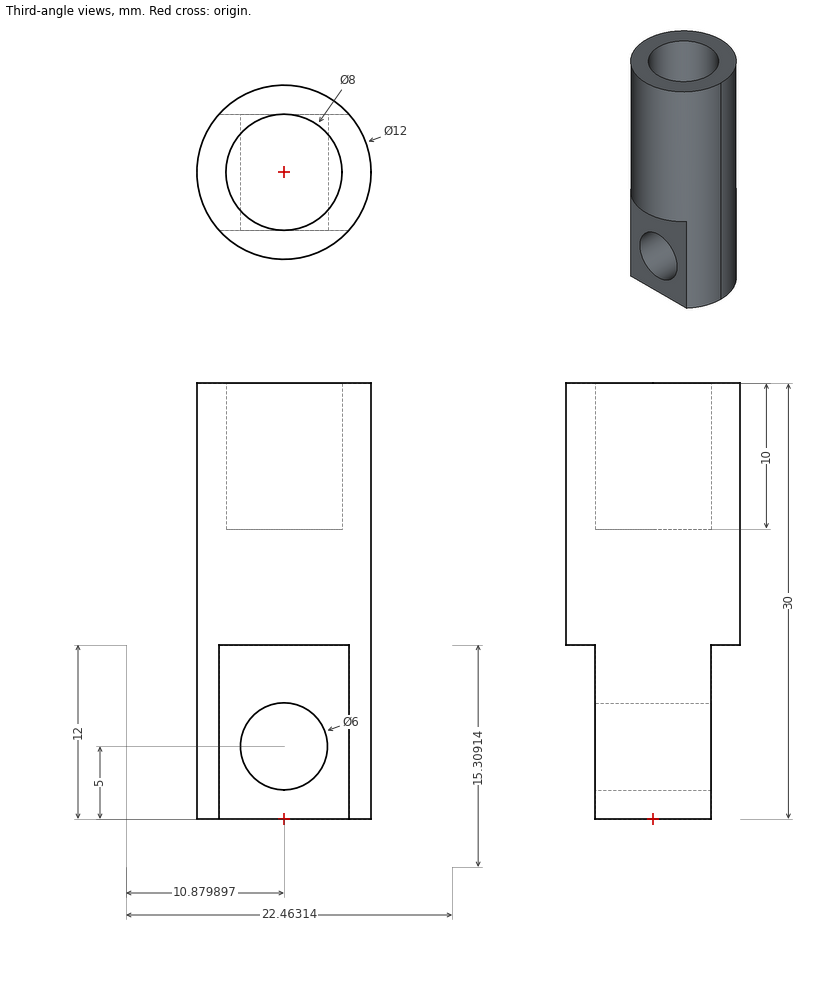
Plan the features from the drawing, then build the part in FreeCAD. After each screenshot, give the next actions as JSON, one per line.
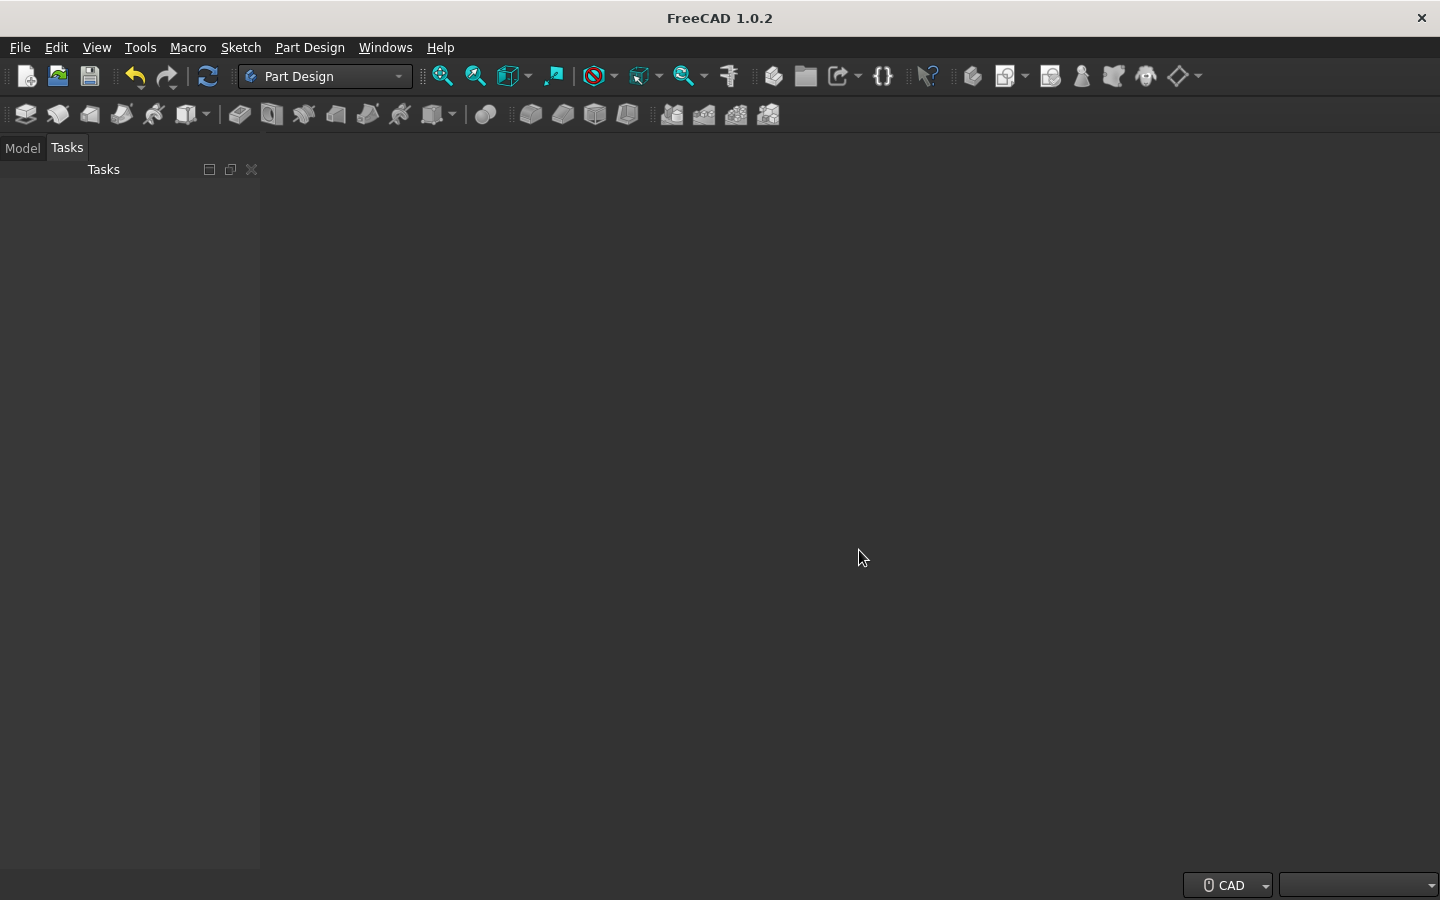
{"action": "left_click", "coordinate": [26, 76]}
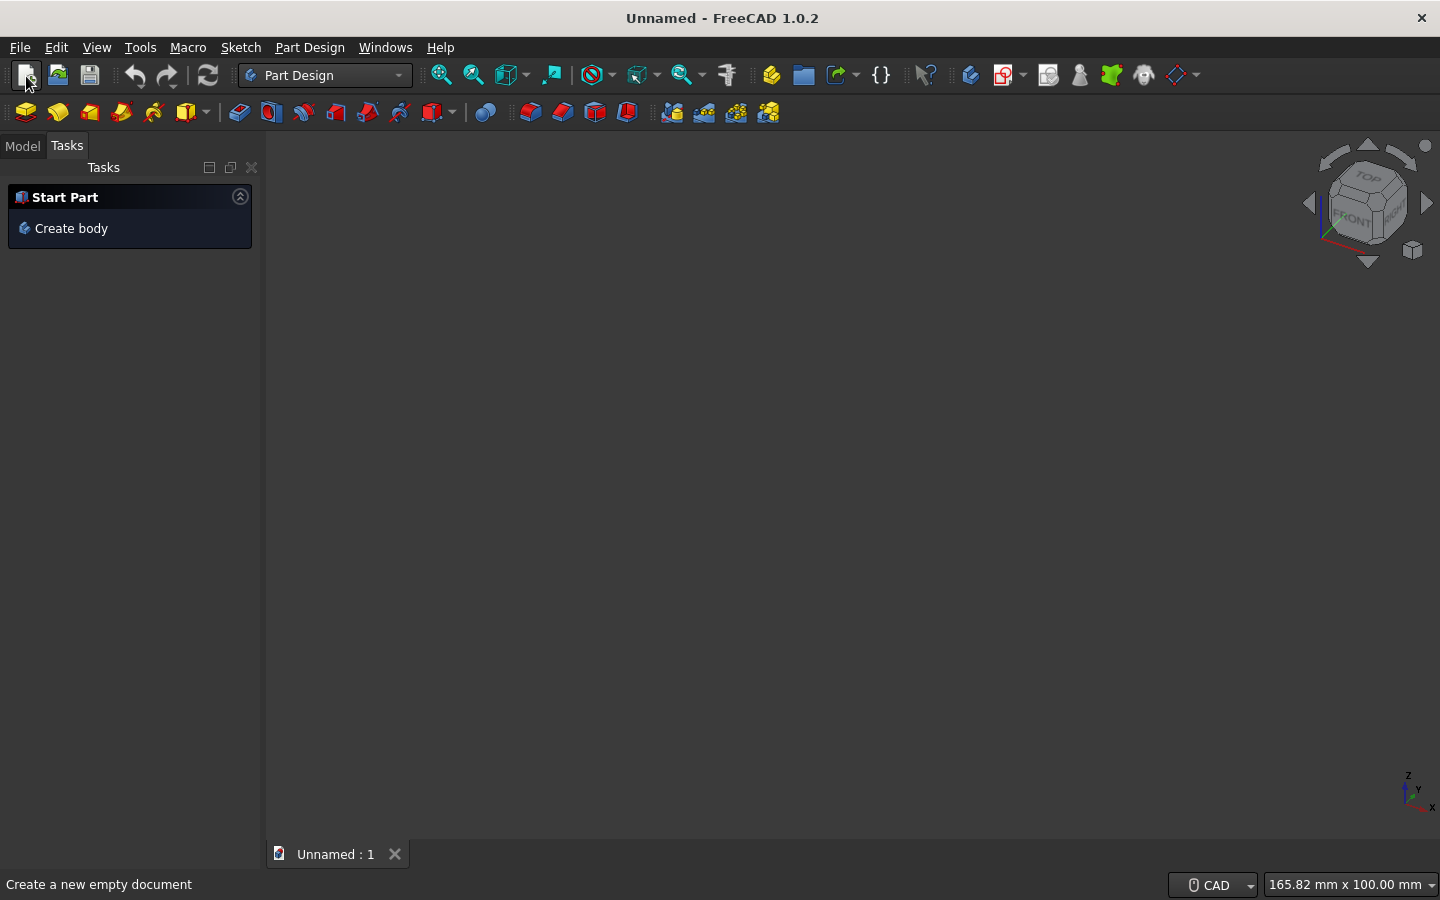
{"action": "left_click", "coordinate": [1004, 76]}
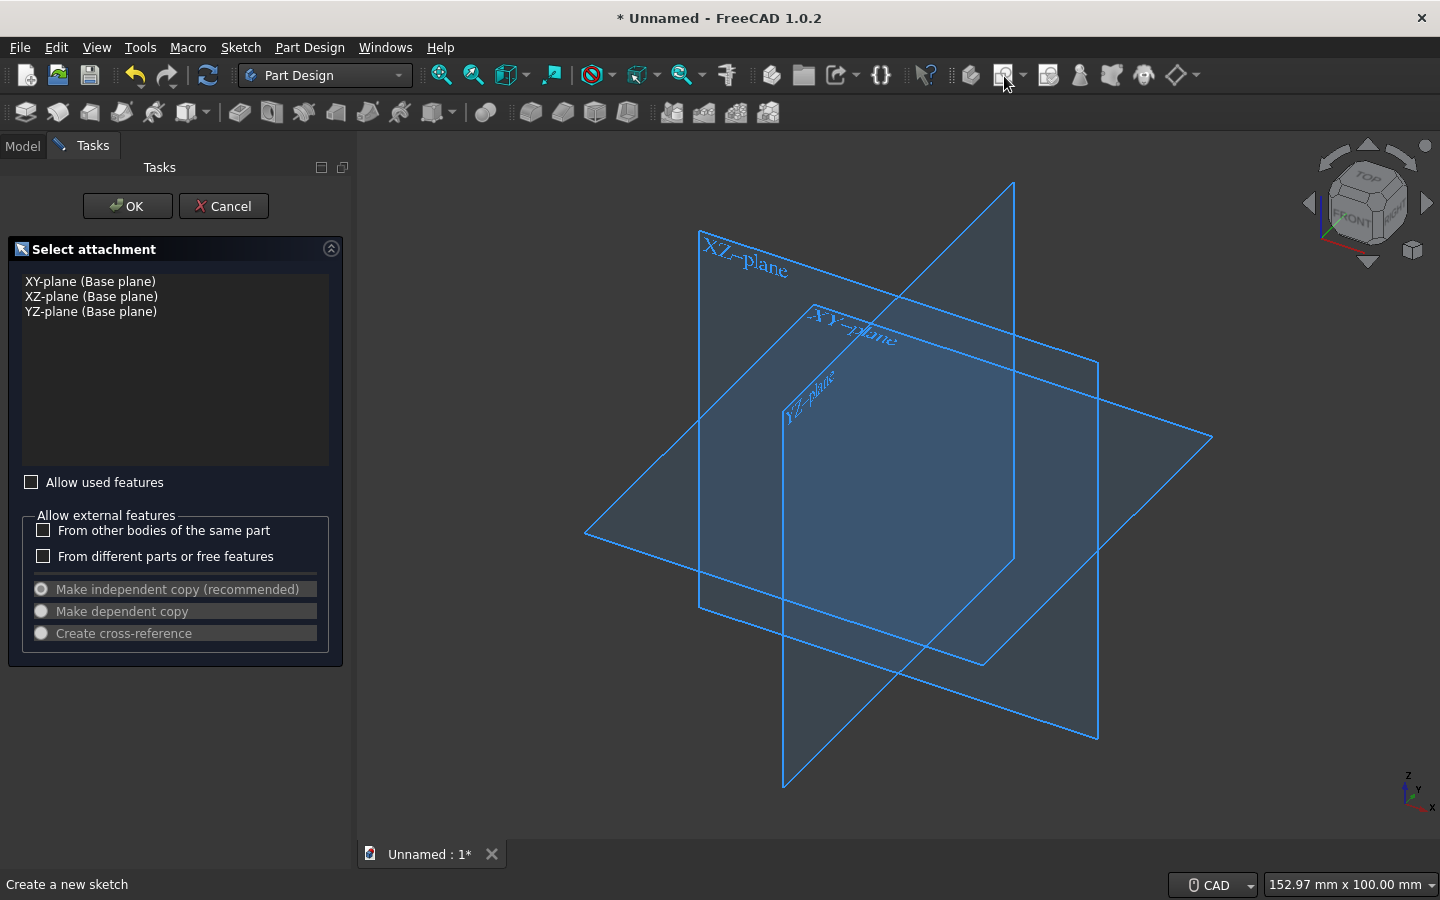
{"action": "left_click", "coordinate": [82, 282]}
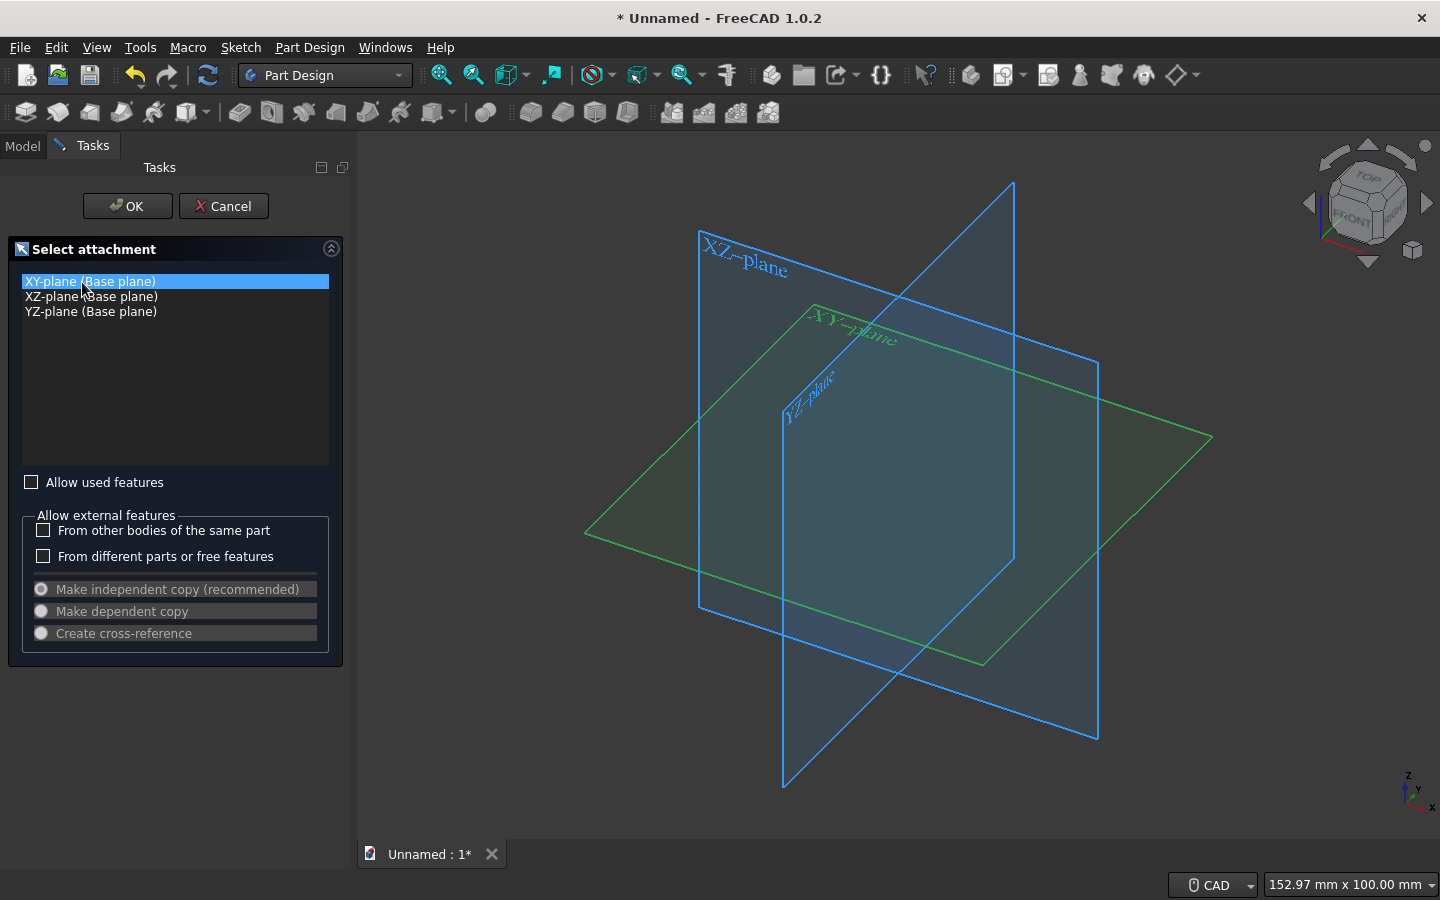
{"action": "left_click", "coordinate": [128, 206]}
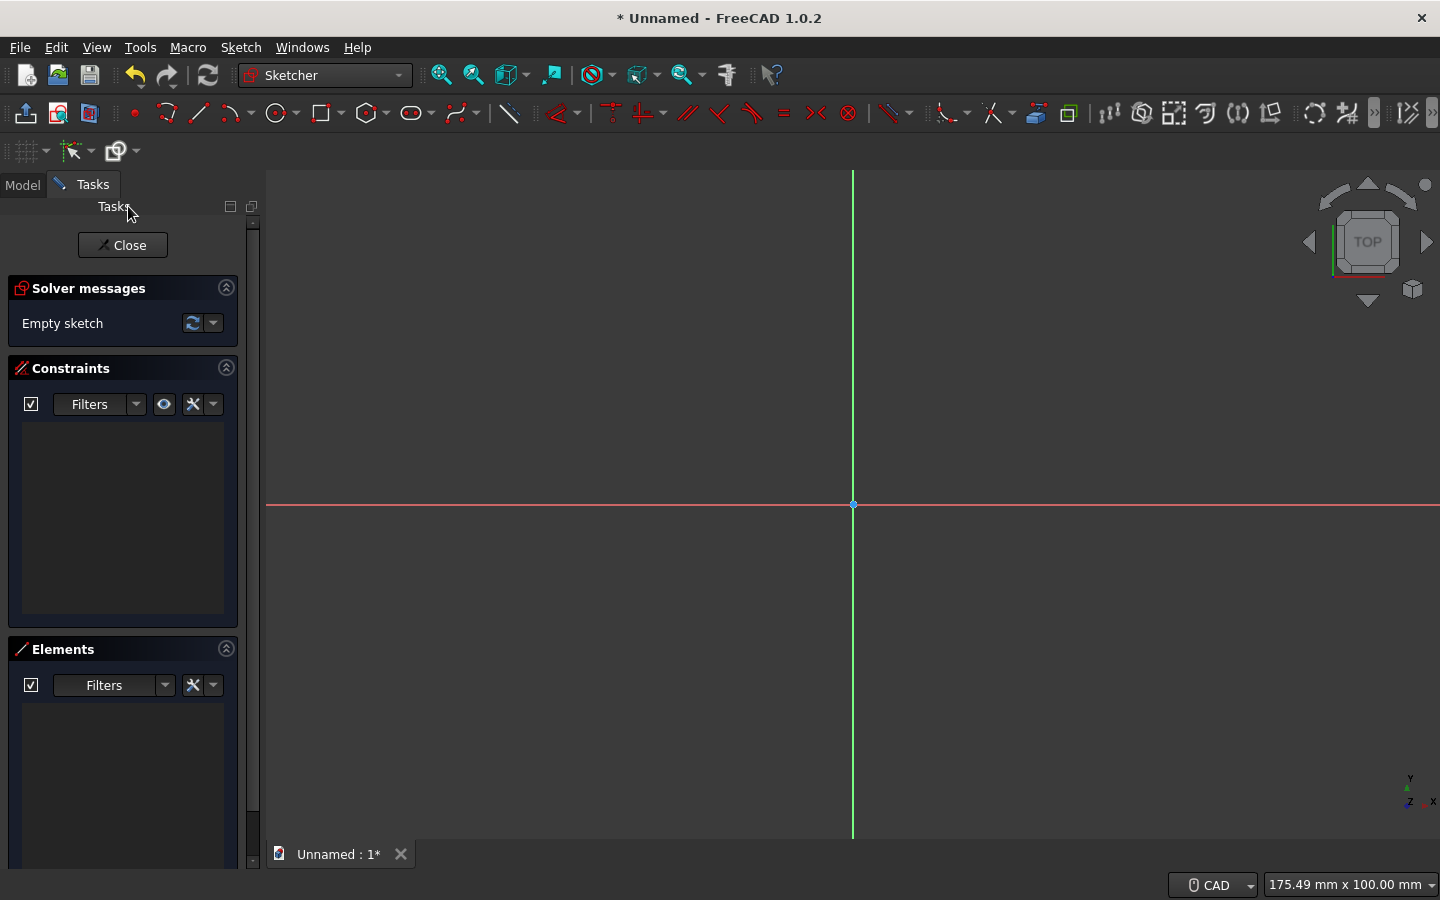
{"action": "scroll", "coordinate": [870, 504], "scroll_direction": "up", "scroll_amount": 8}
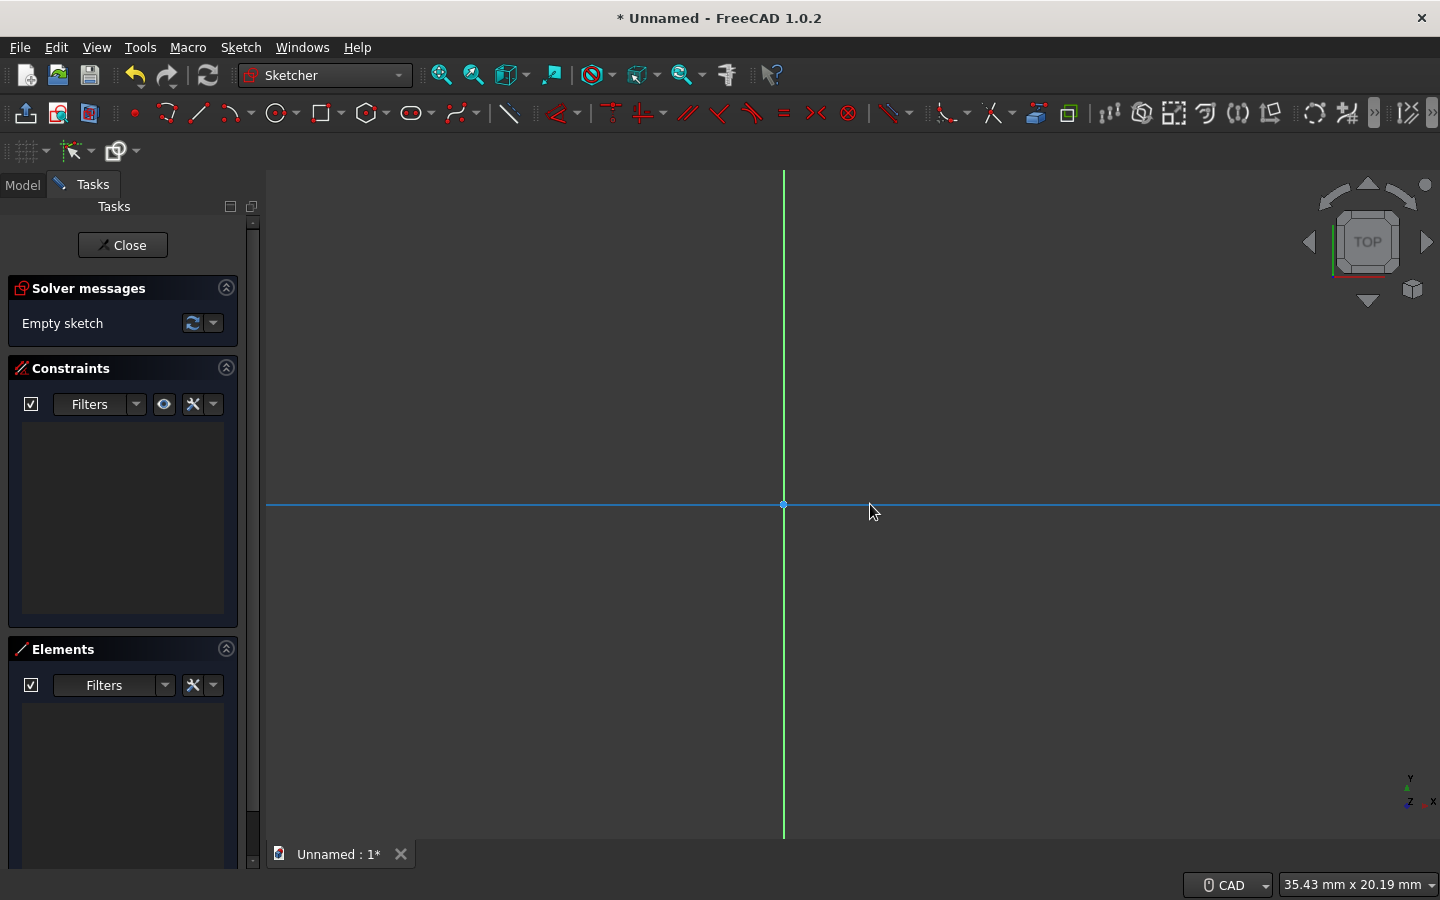
{"action": "left_click", "coordinate": [276, 114]}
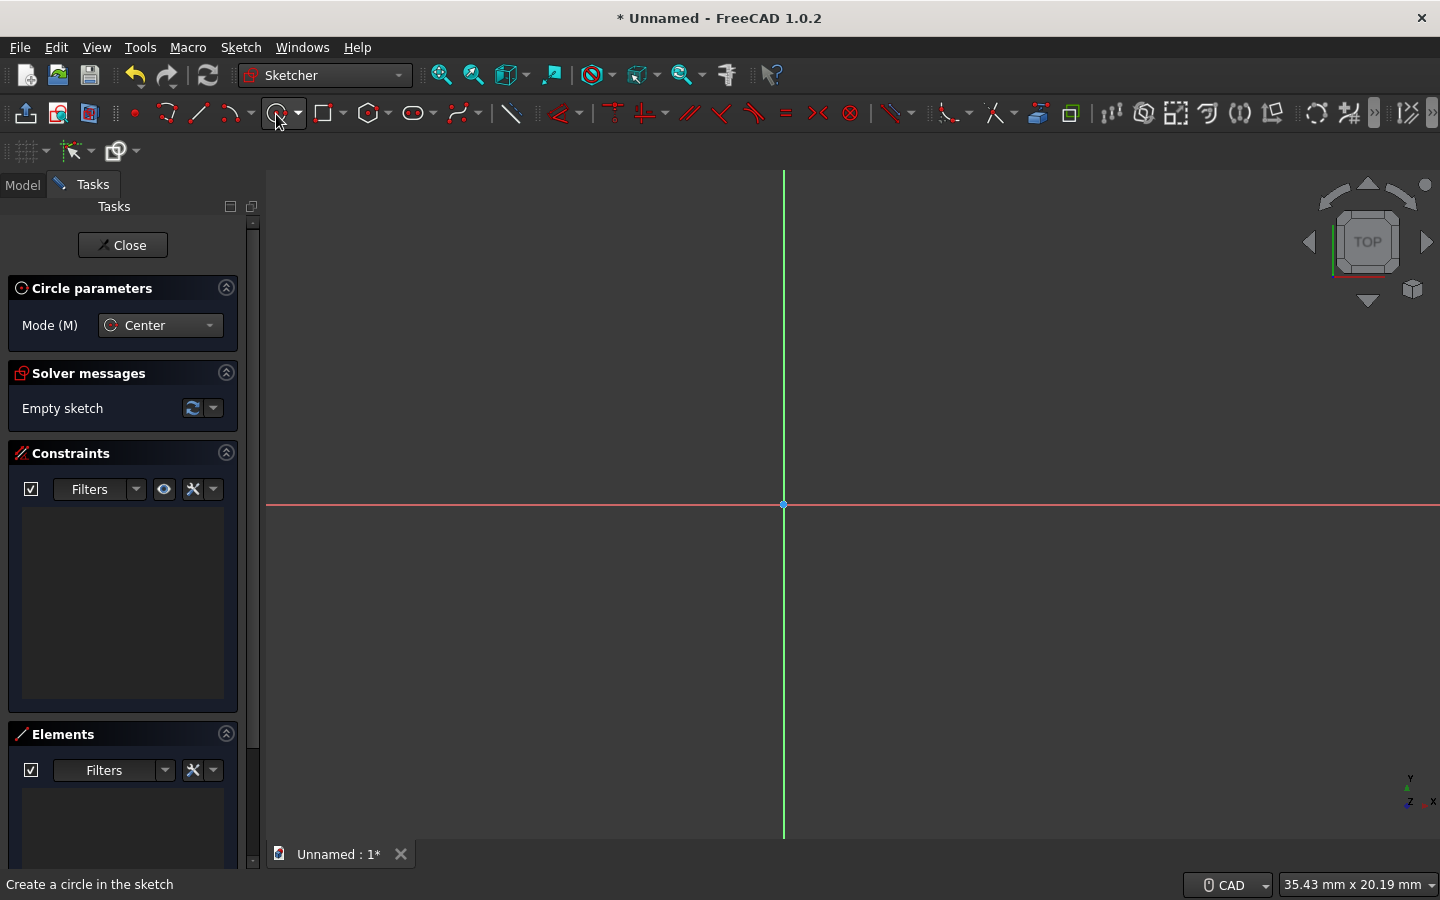
{"action": "left_click", "coordinate": [784, 504]}
{"action": "mouse_move", "coordinate": [924, 364]}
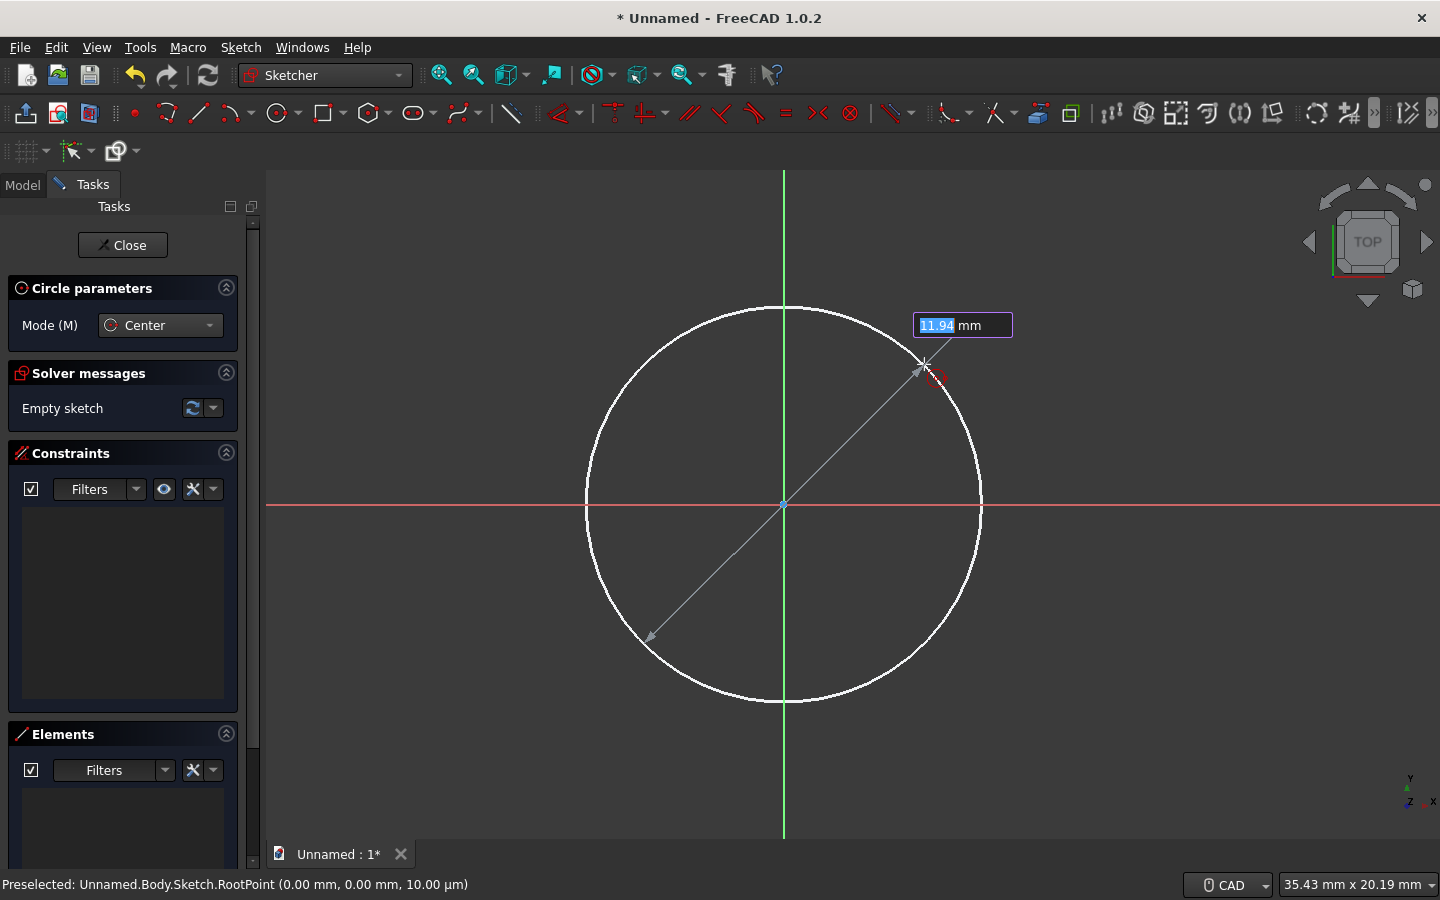
{"action": "type", "text": "12"}
{"action": "key", "text": "Return"}
{"action": "key", "text": "Escape"}